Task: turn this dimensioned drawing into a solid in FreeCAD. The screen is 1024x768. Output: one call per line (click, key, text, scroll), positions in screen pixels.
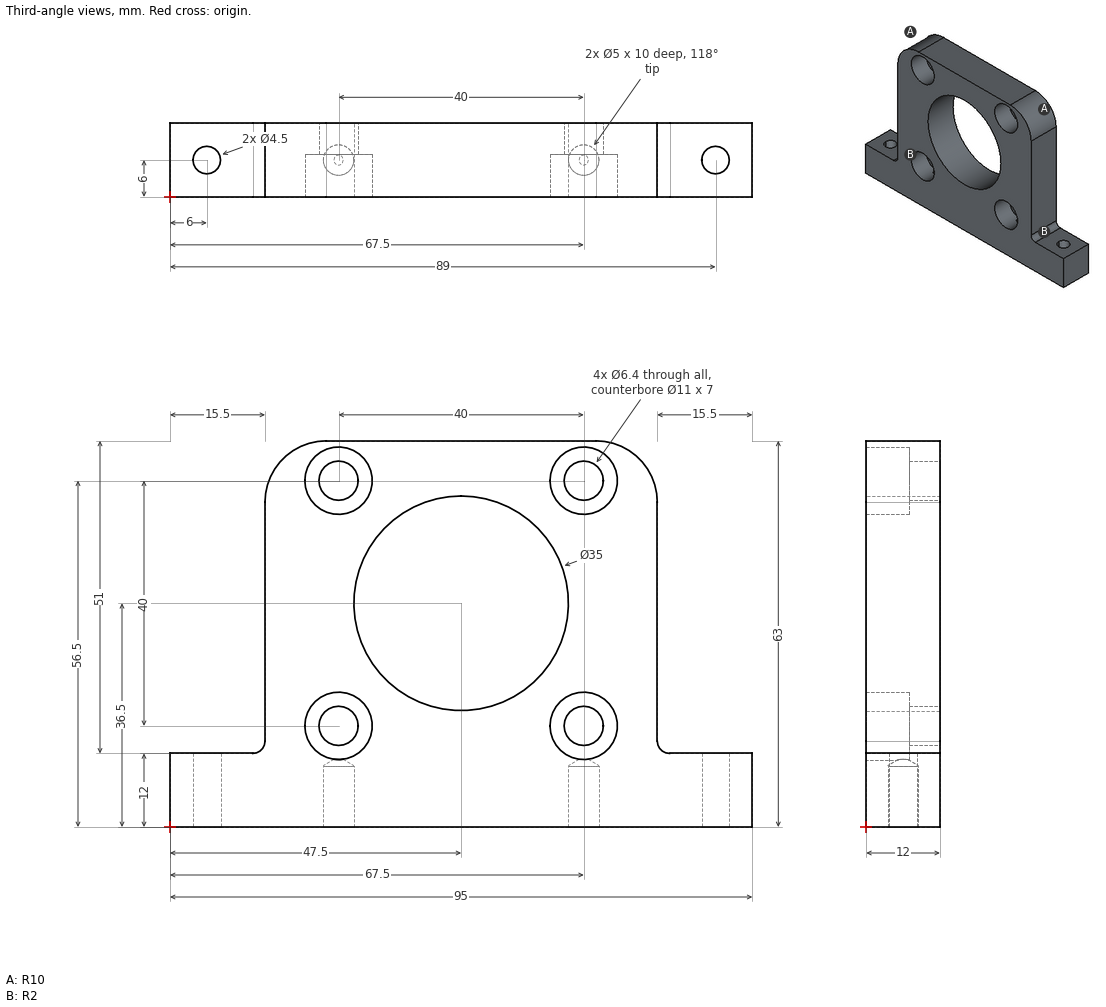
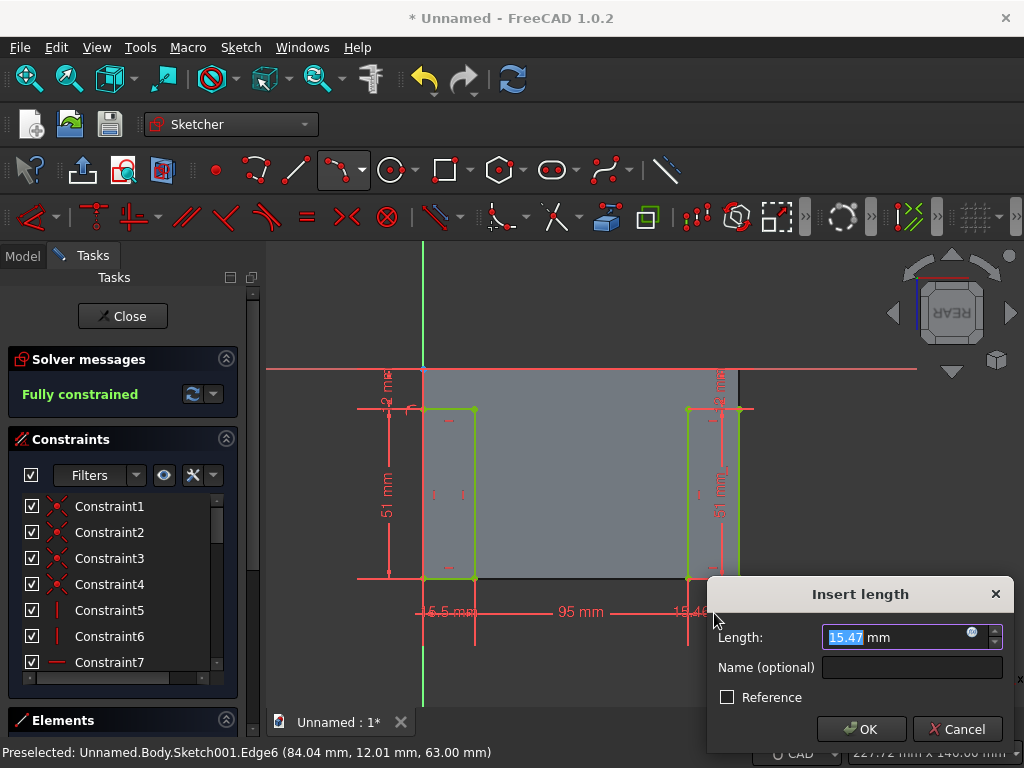
text(15.5)
key(Return)
key(Escape)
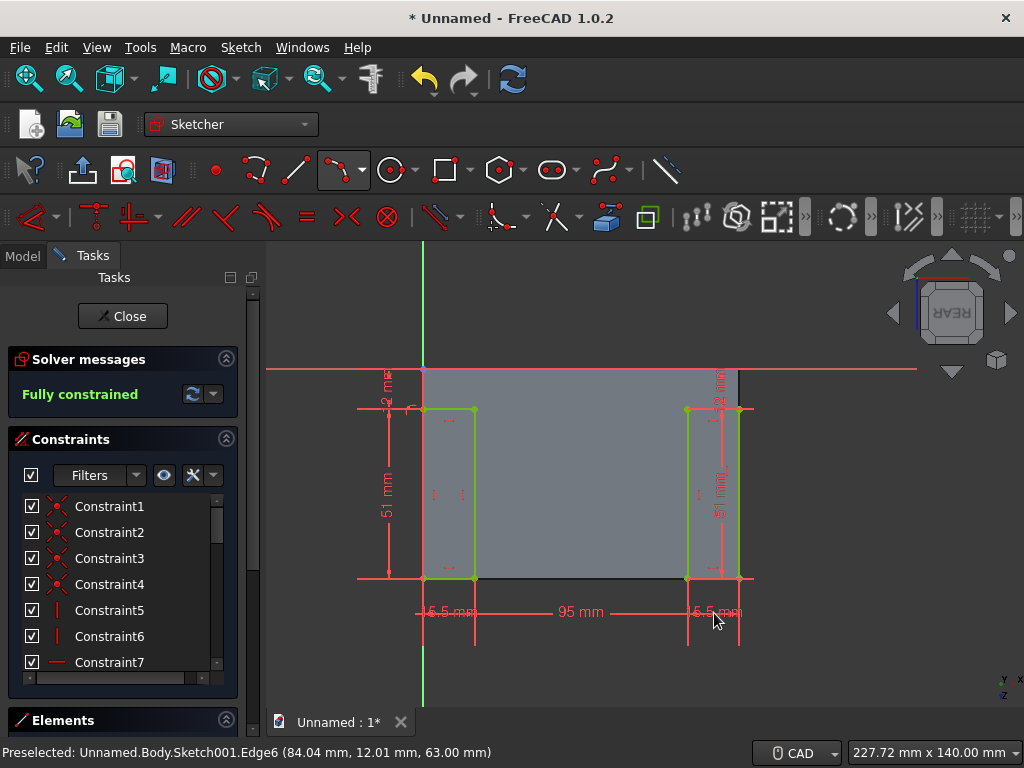
click(123, 316)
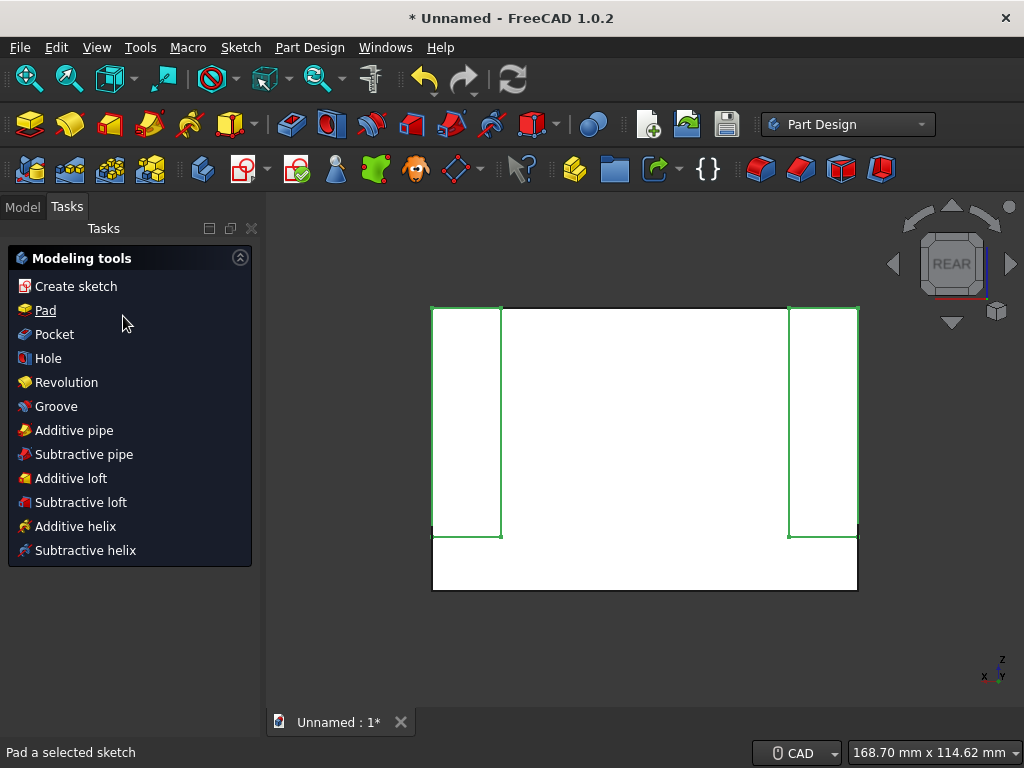
click(292, 124)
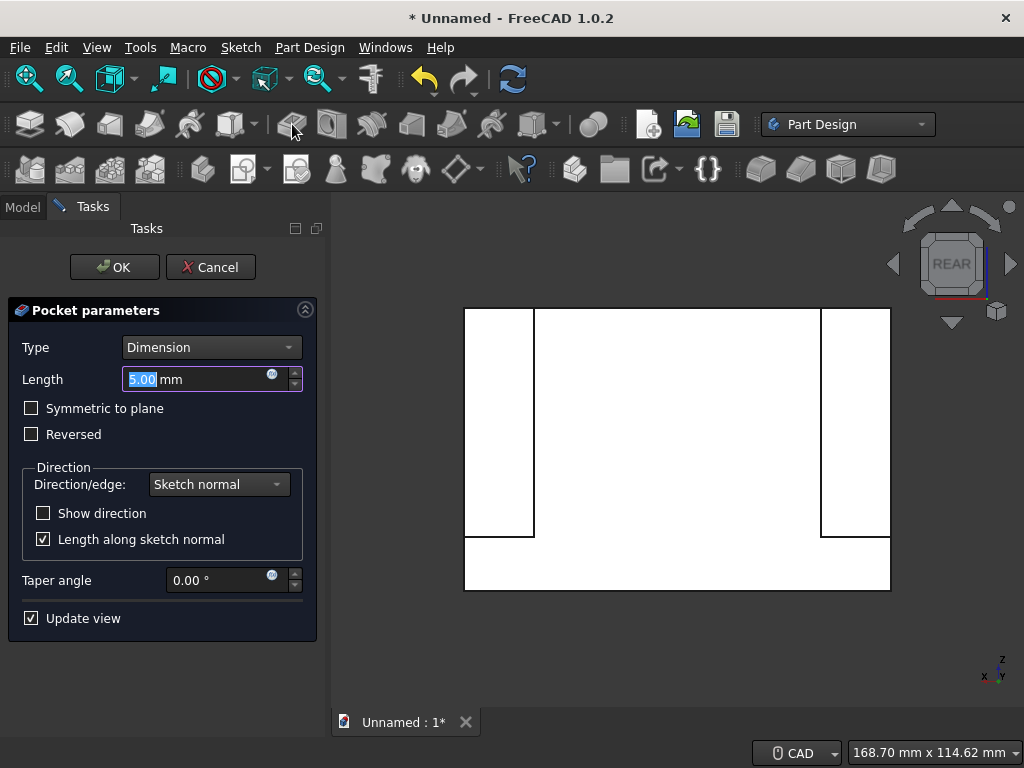
click(212, 348)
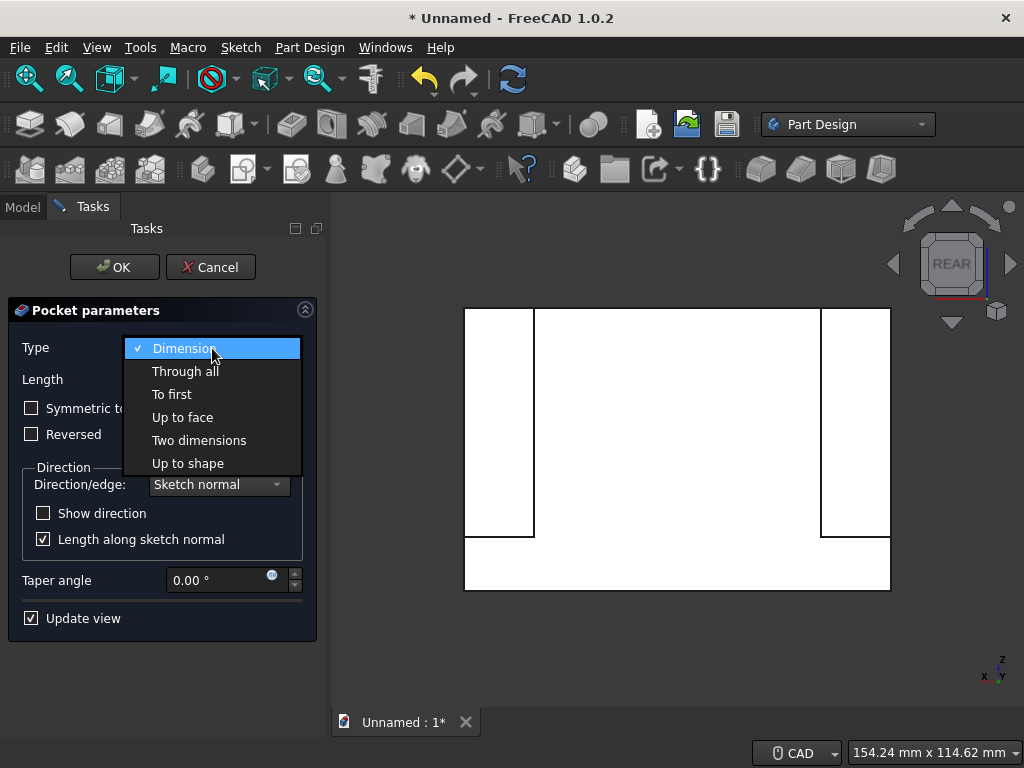
click(212, 372)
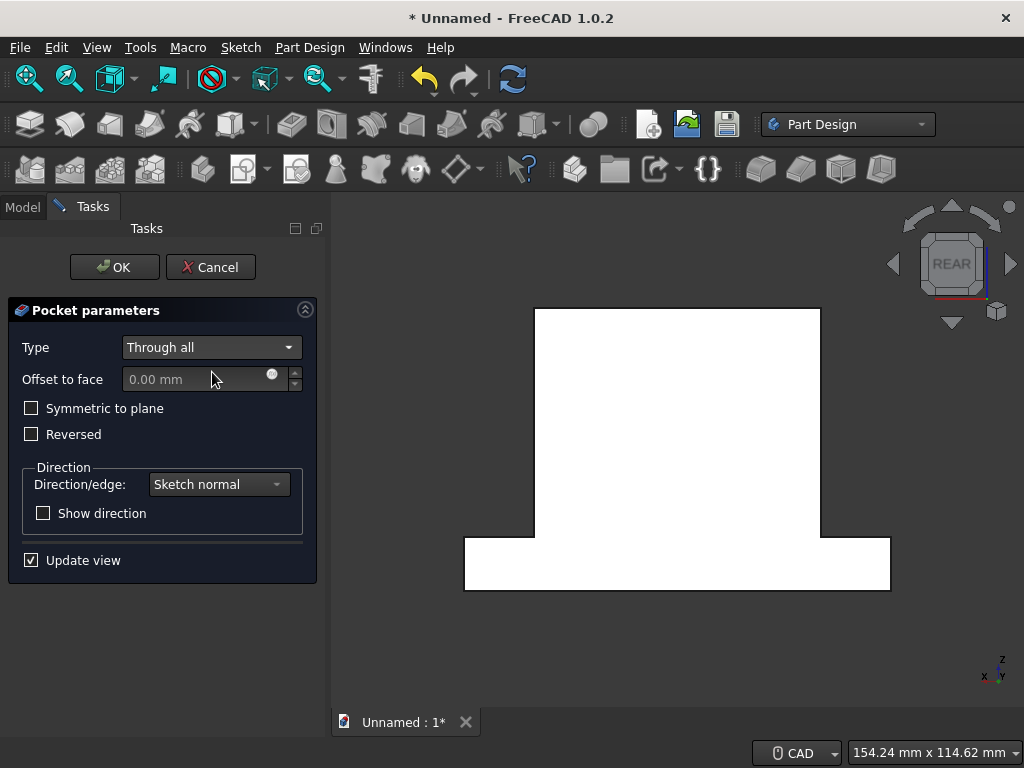
click(115, 267)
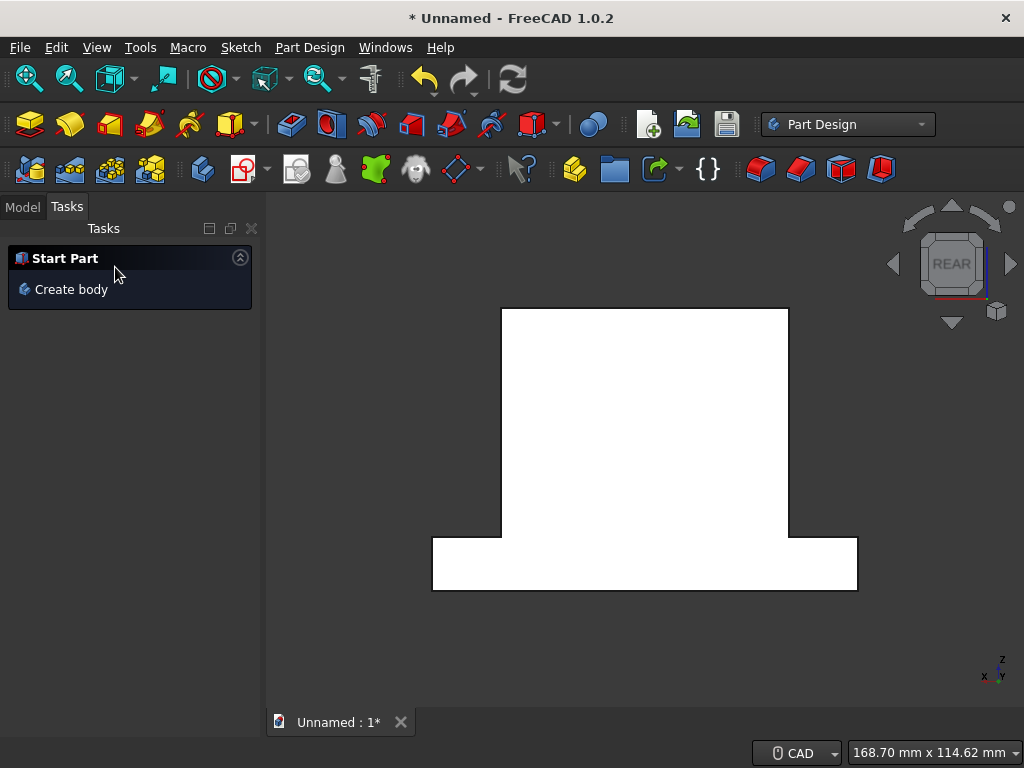
key(0)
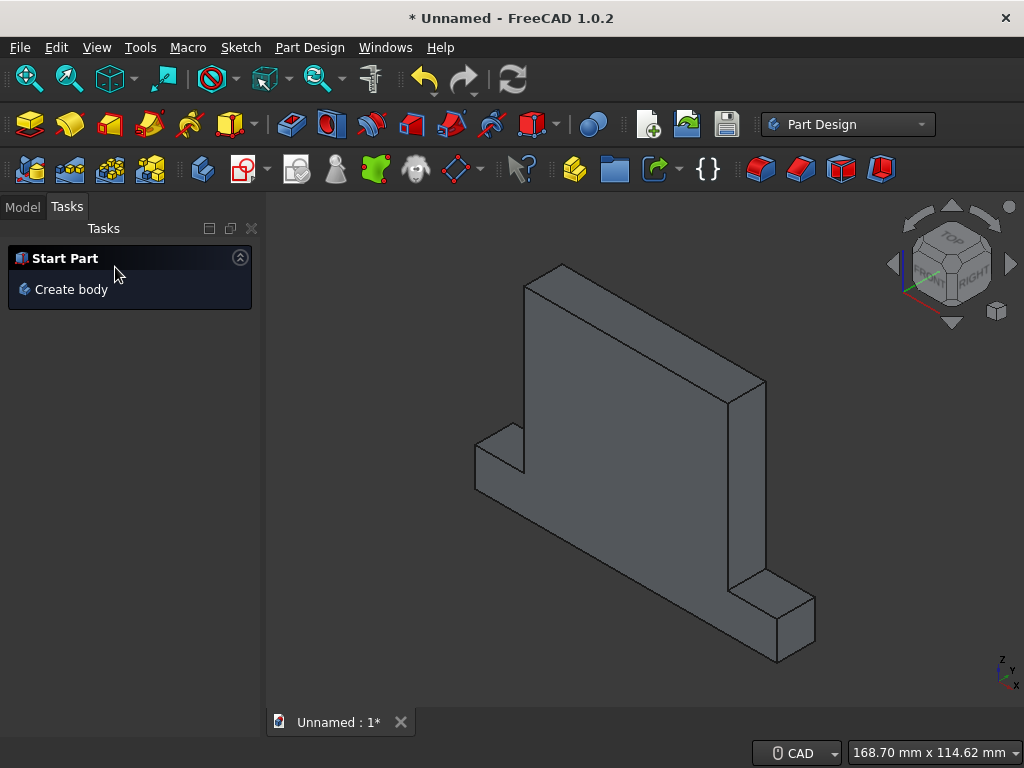
click(512, 443)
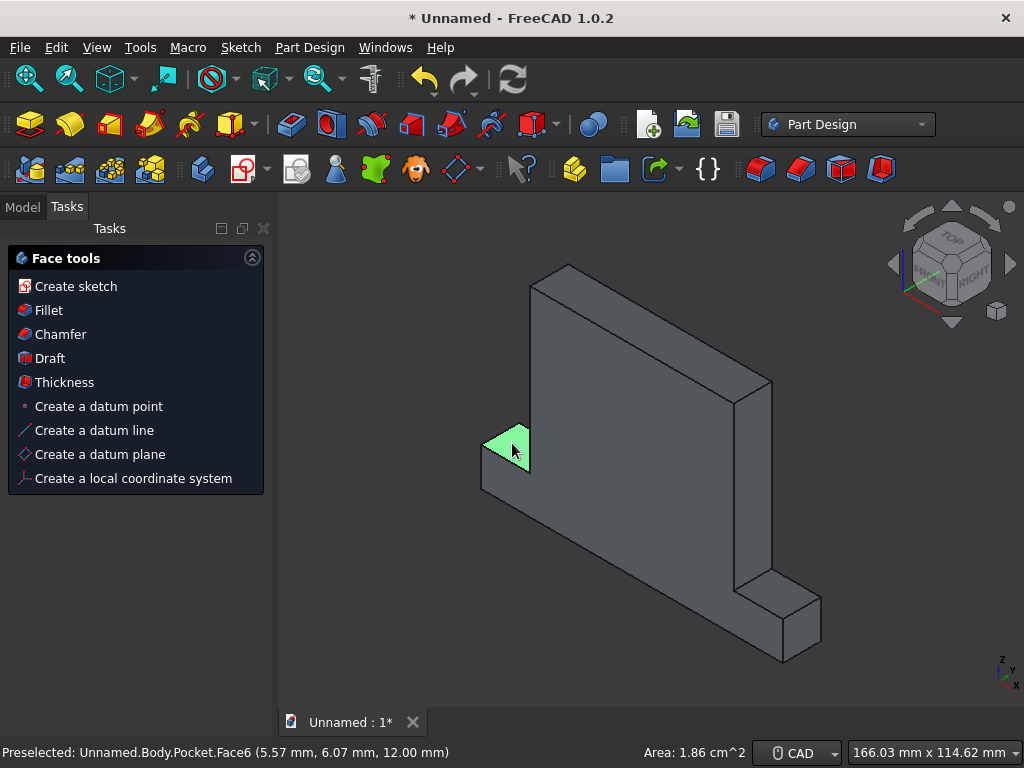
click(244, 170)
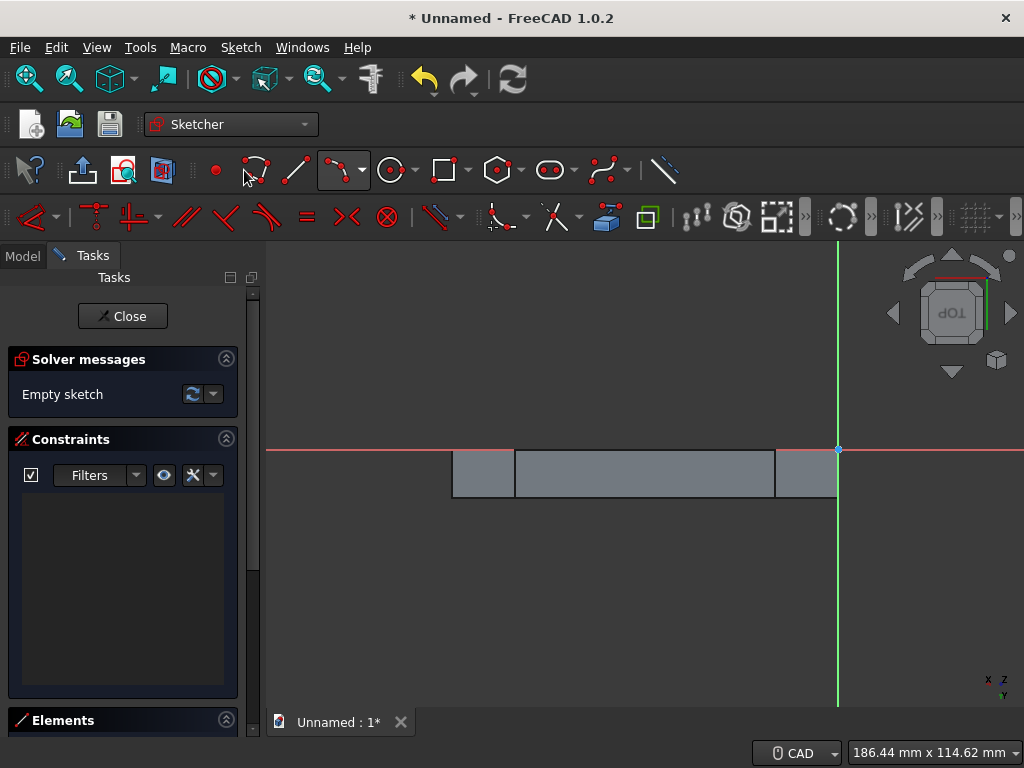
click(164, 170)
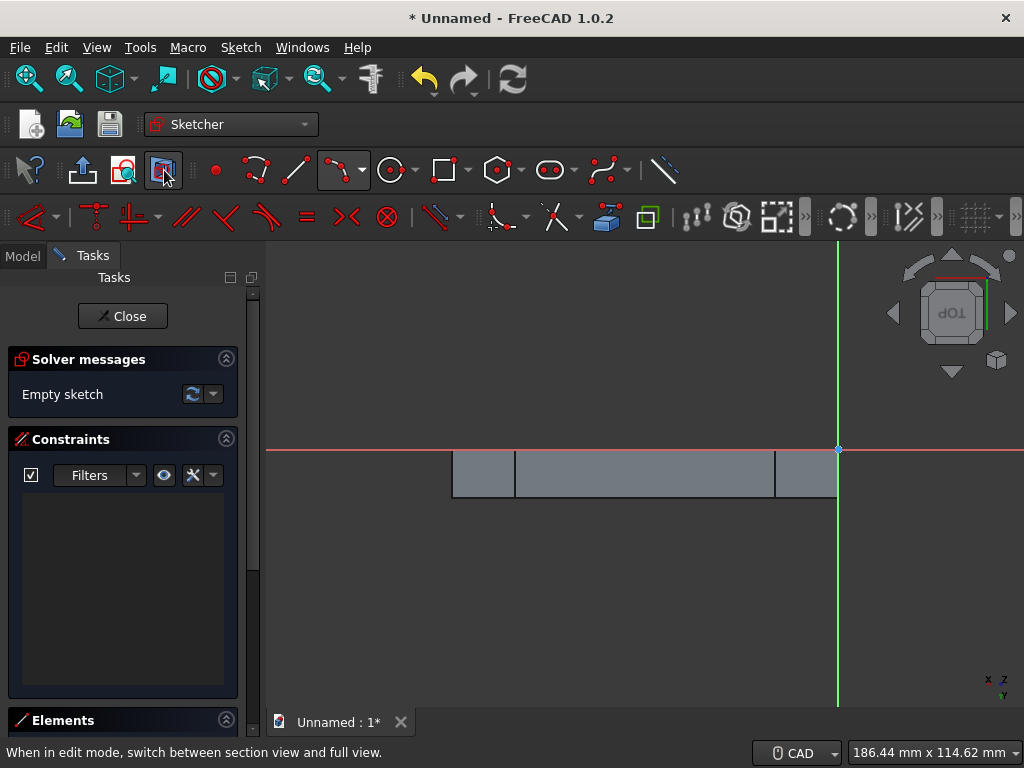
scroll(294, 508, down, 1)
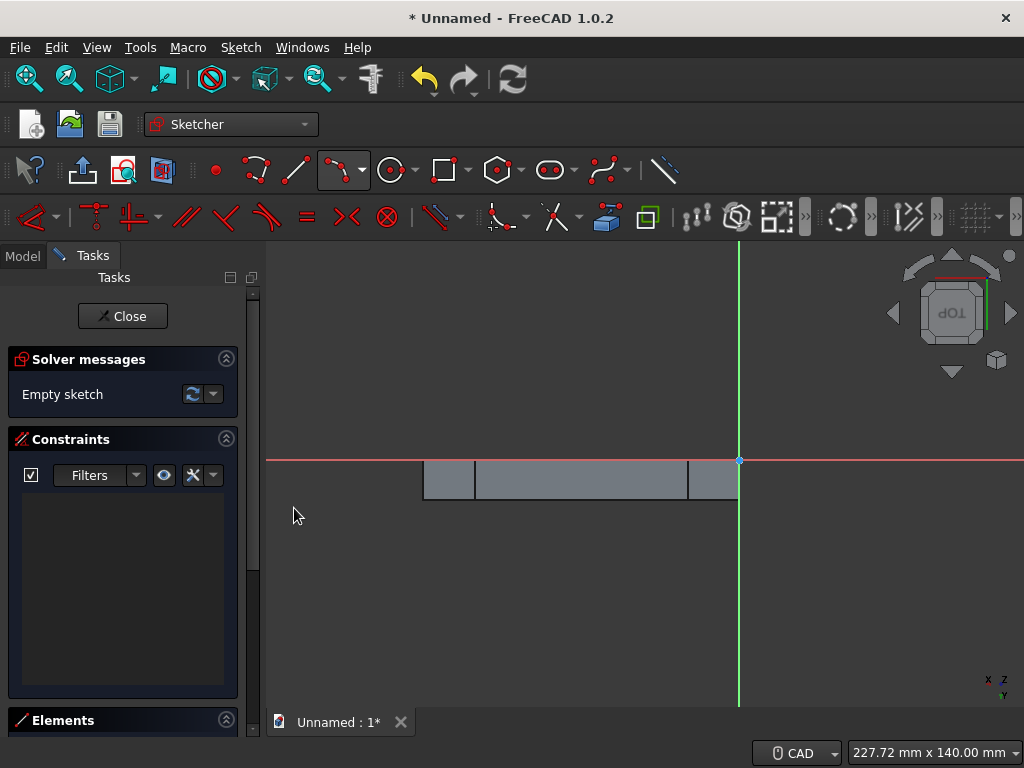
key(g)
key(c)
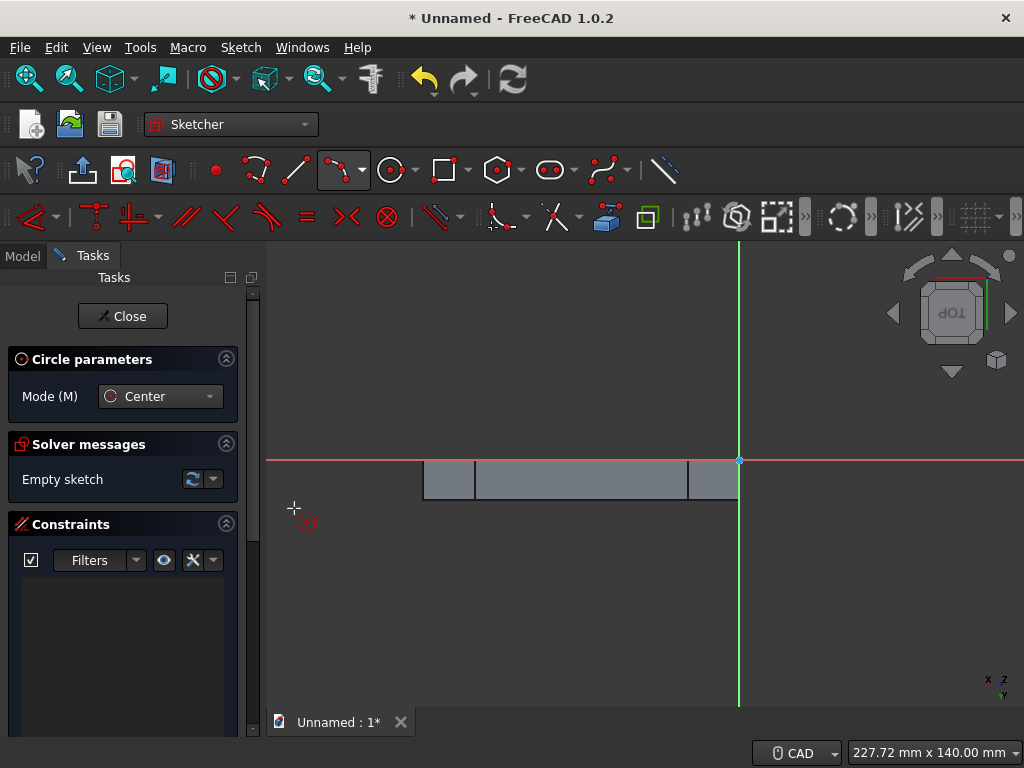
scroll(720, 480, up, 6)